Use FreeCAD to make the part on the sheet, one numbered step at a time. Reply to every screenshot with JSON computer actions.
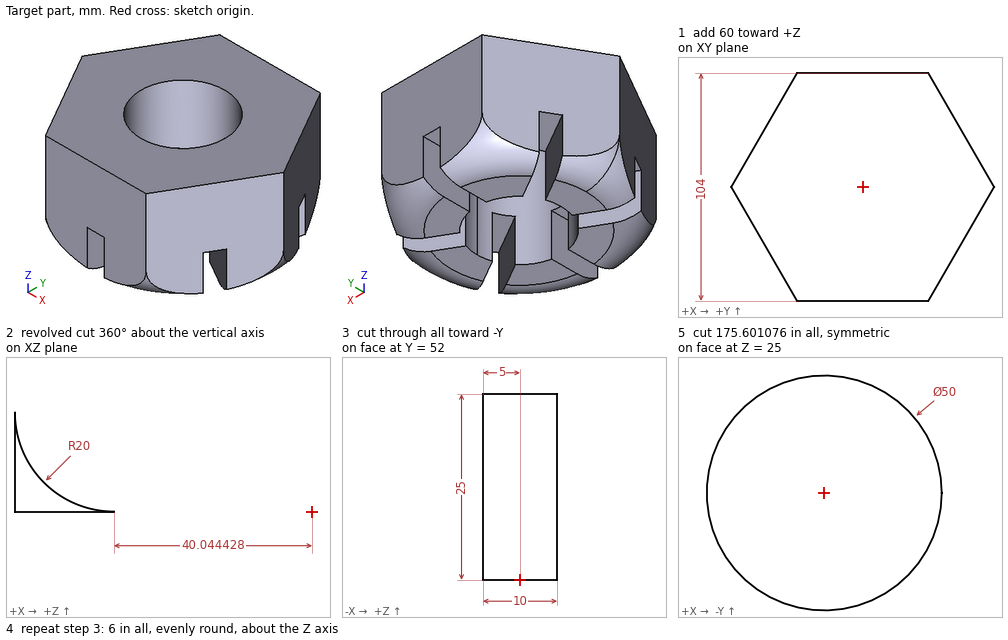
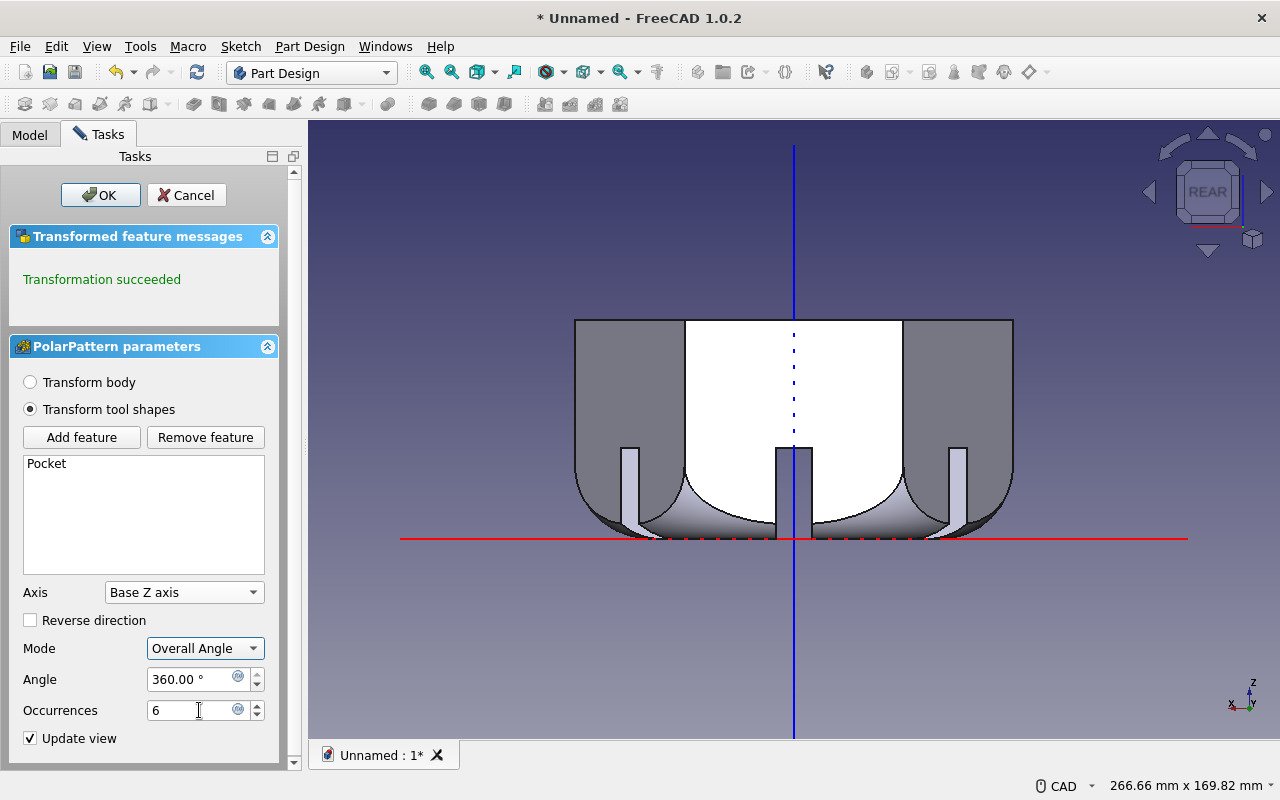
{"action": "left_click", "coordinate": [101, 195]}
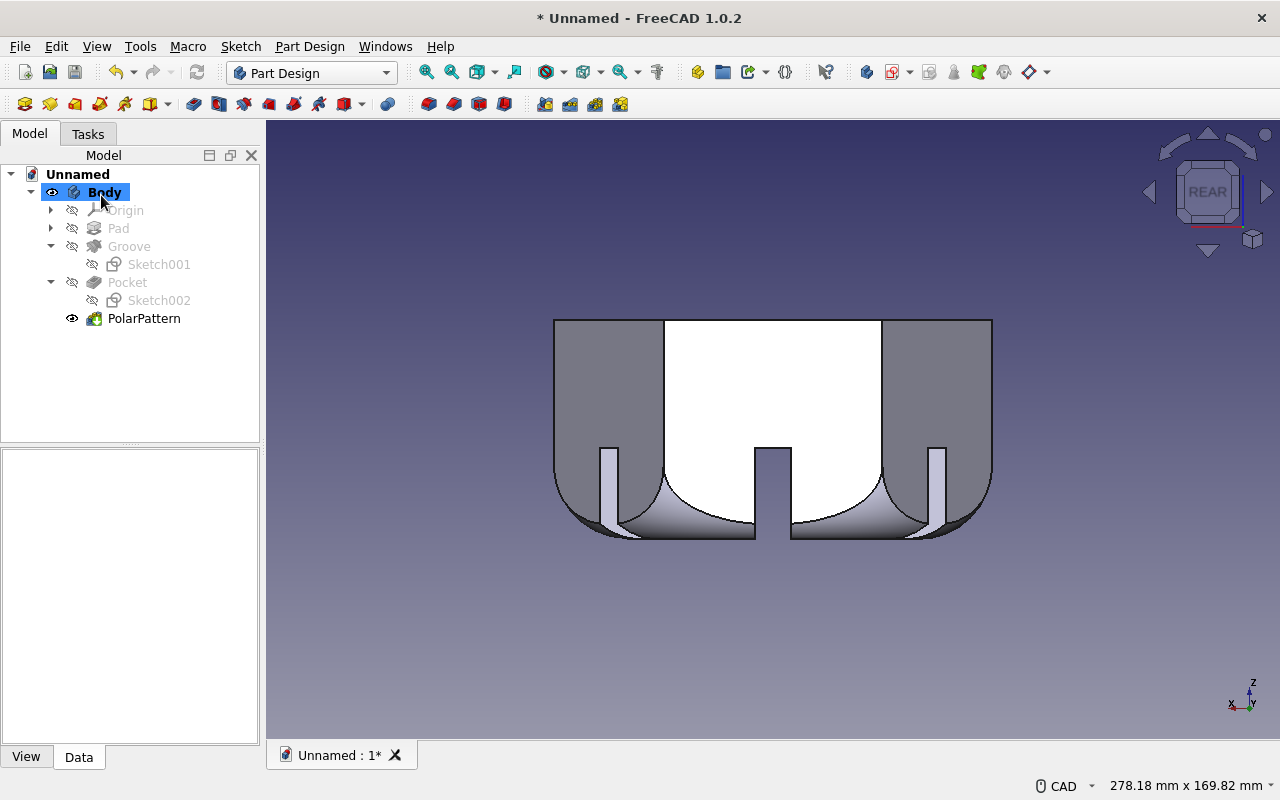
{"action": "left_click", "coordinate": [427, 72]}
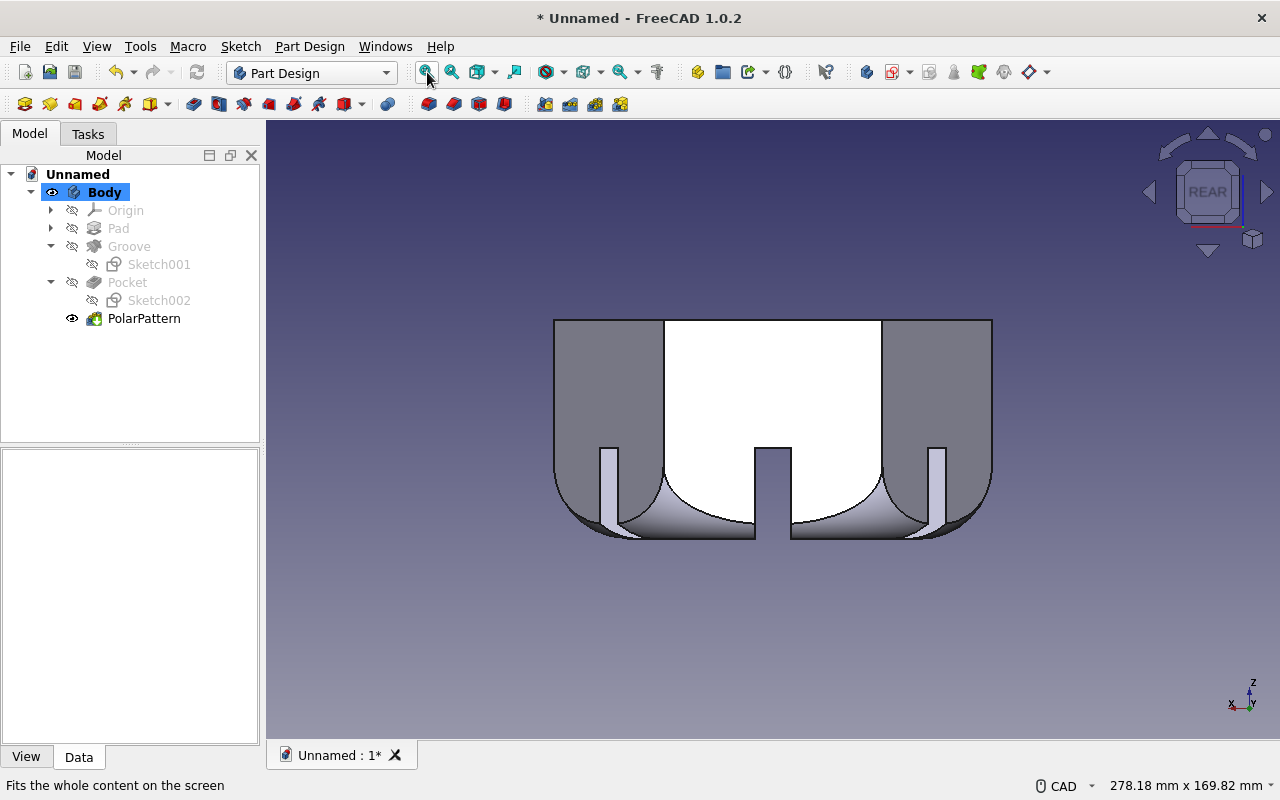
{"action": "key", "text": "5"}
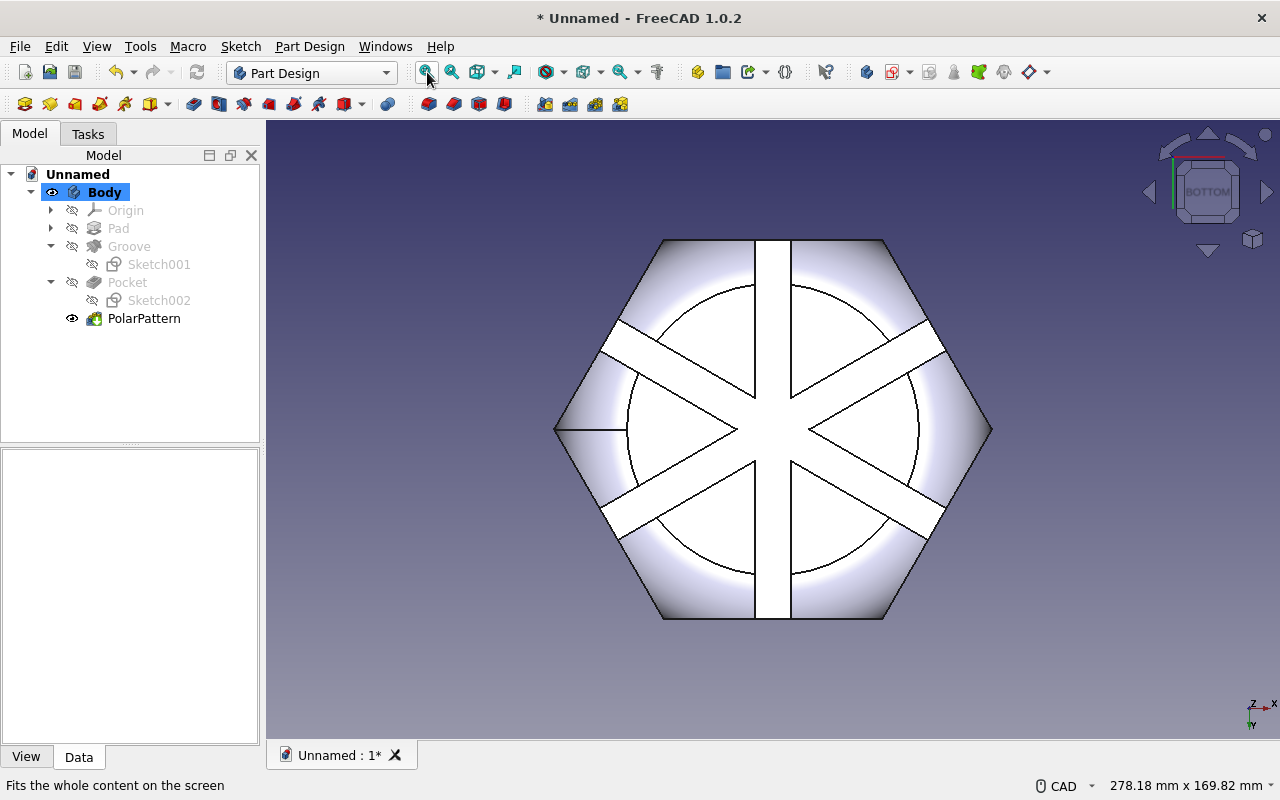
{"action": "left_click", "coordinate": [773, 428]}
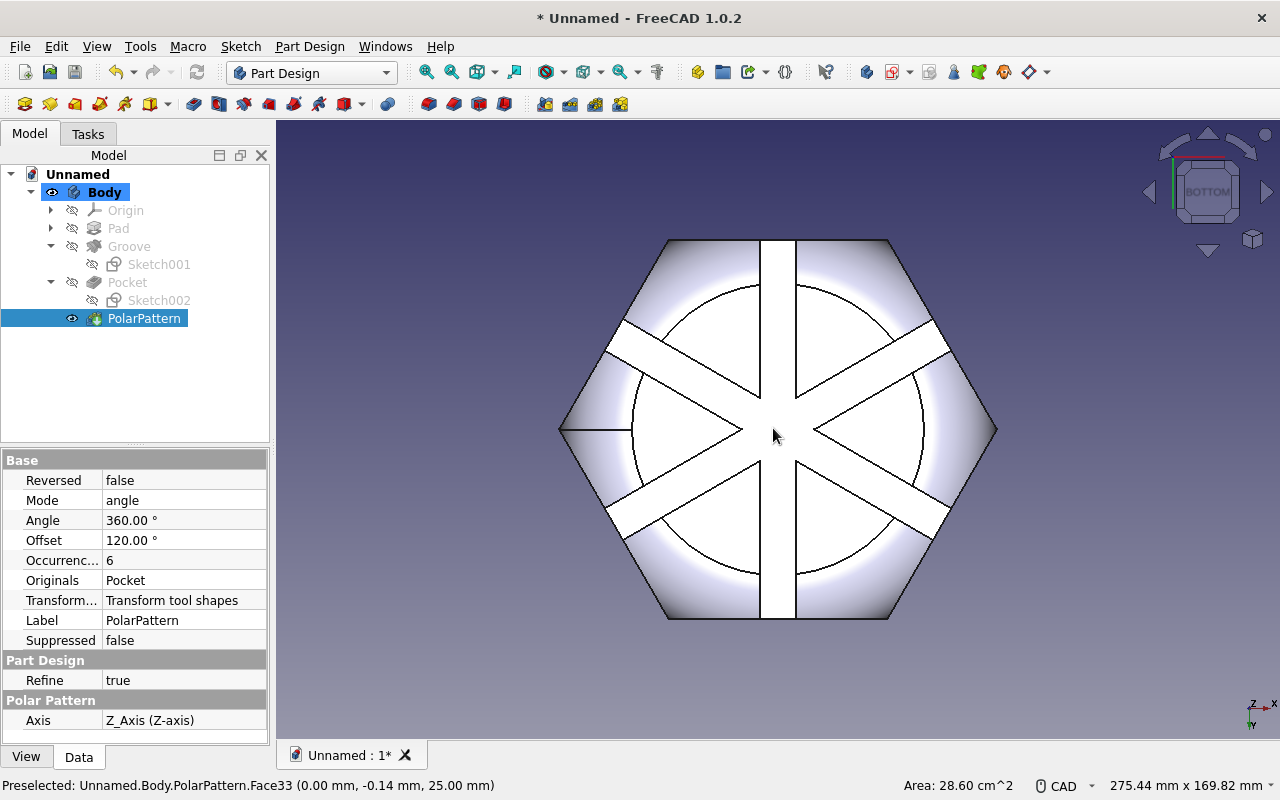
{"action": "left_click", "coordinate": [892, 72]}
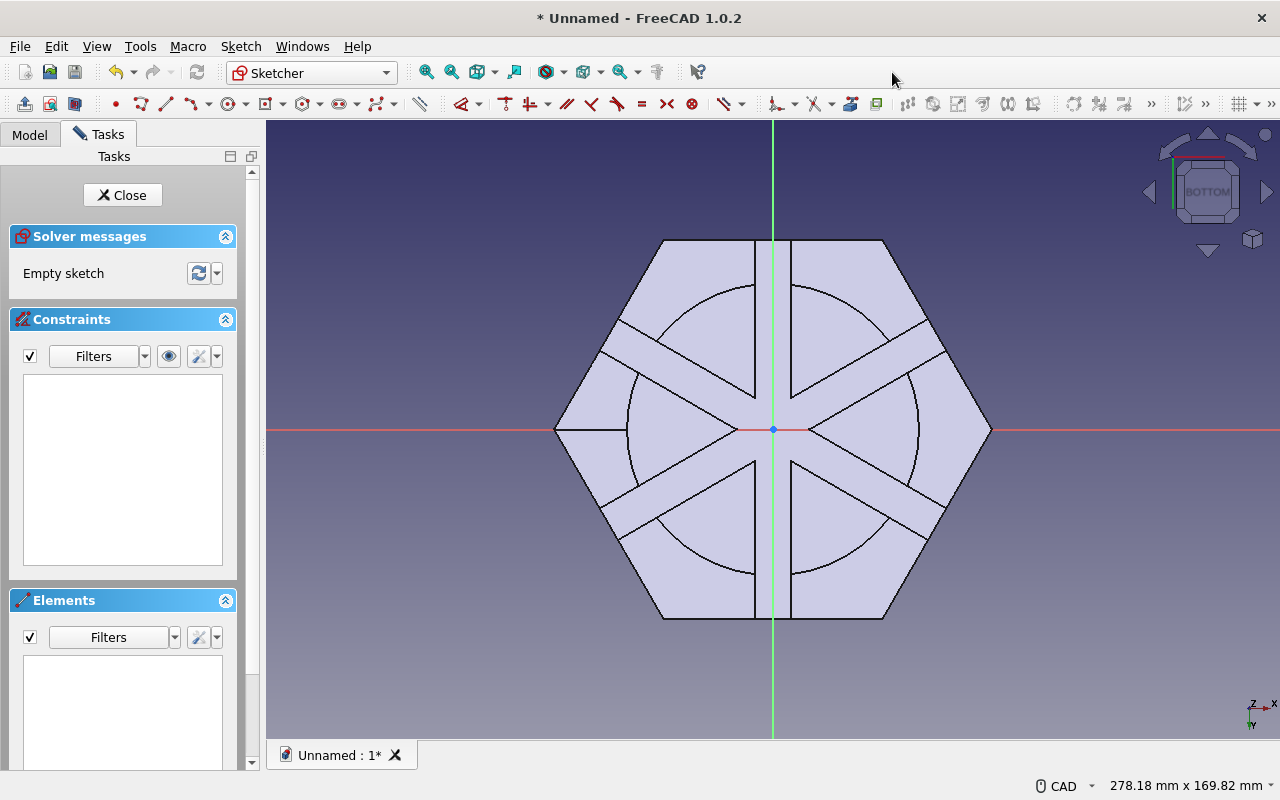
{"action": "key", "text": "q s"}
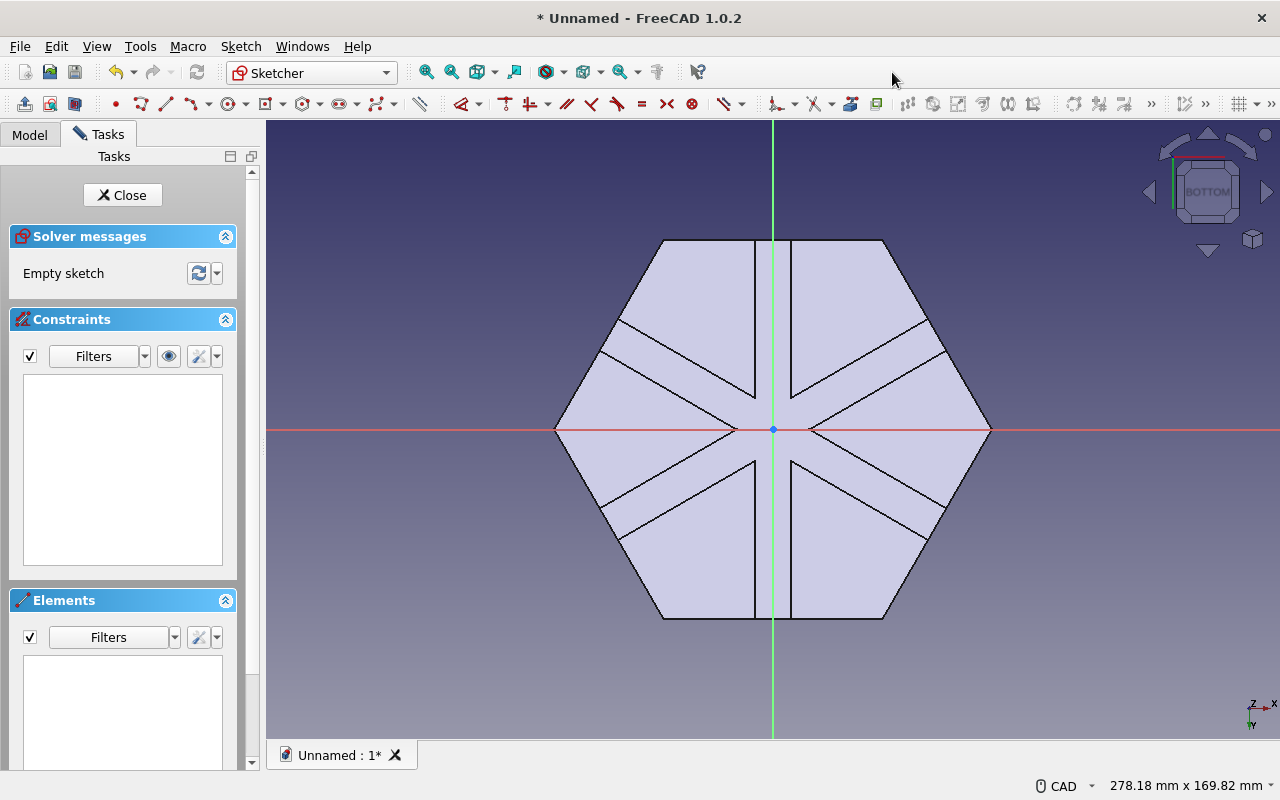
{"action": "scroll", "coordinate": [829, 430], "scroll_direction": "up", "scroll_amount": 4}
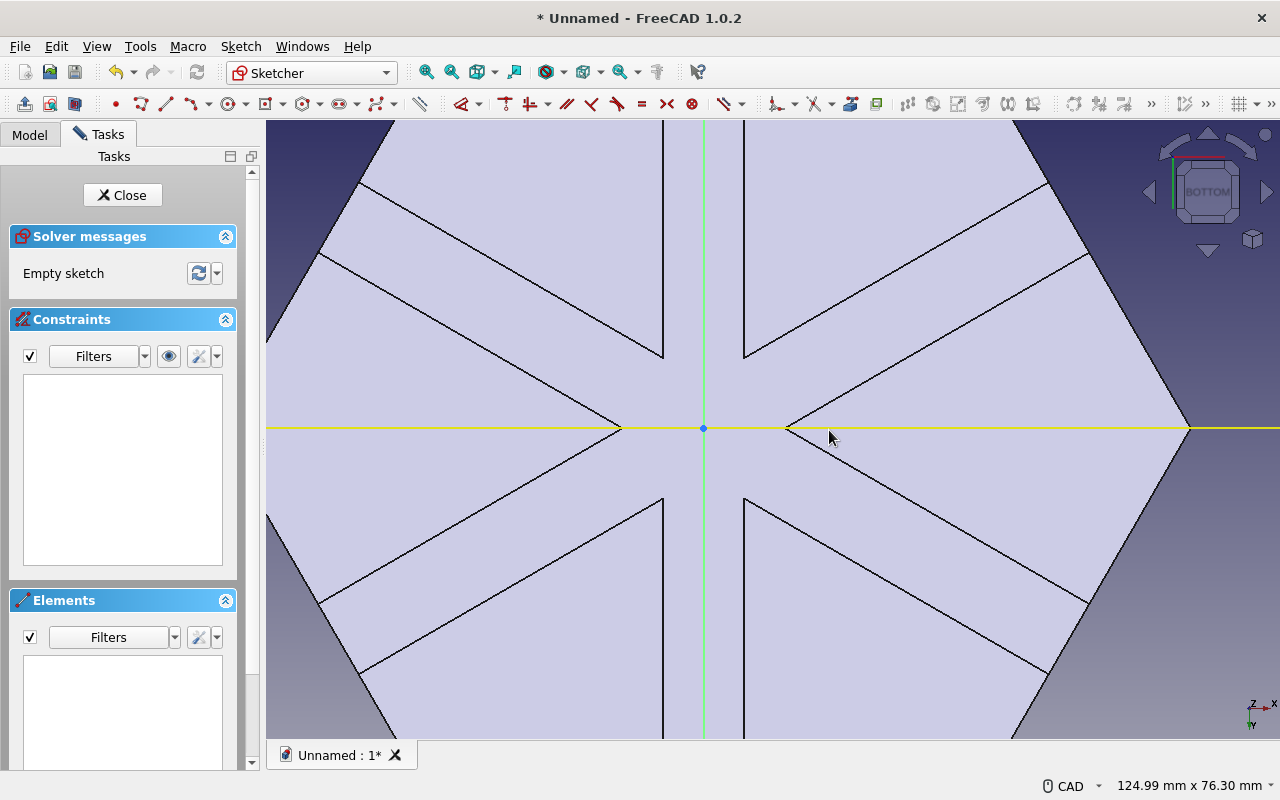
{"action": "left_click", "coordinate": [228, 104]}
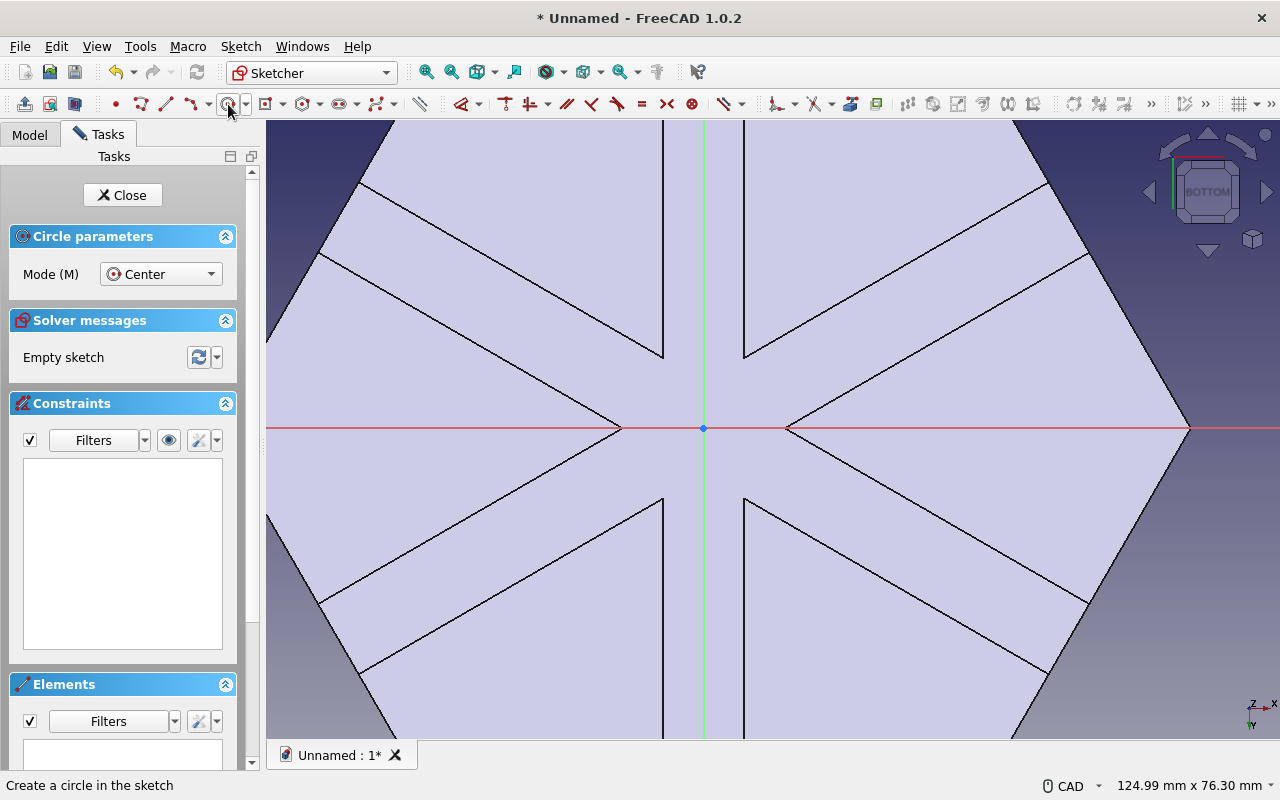
{"action": "left_click", "coordinate": [704, 428]}
{"action": "mouse_move", "coordinate": [847, 285]}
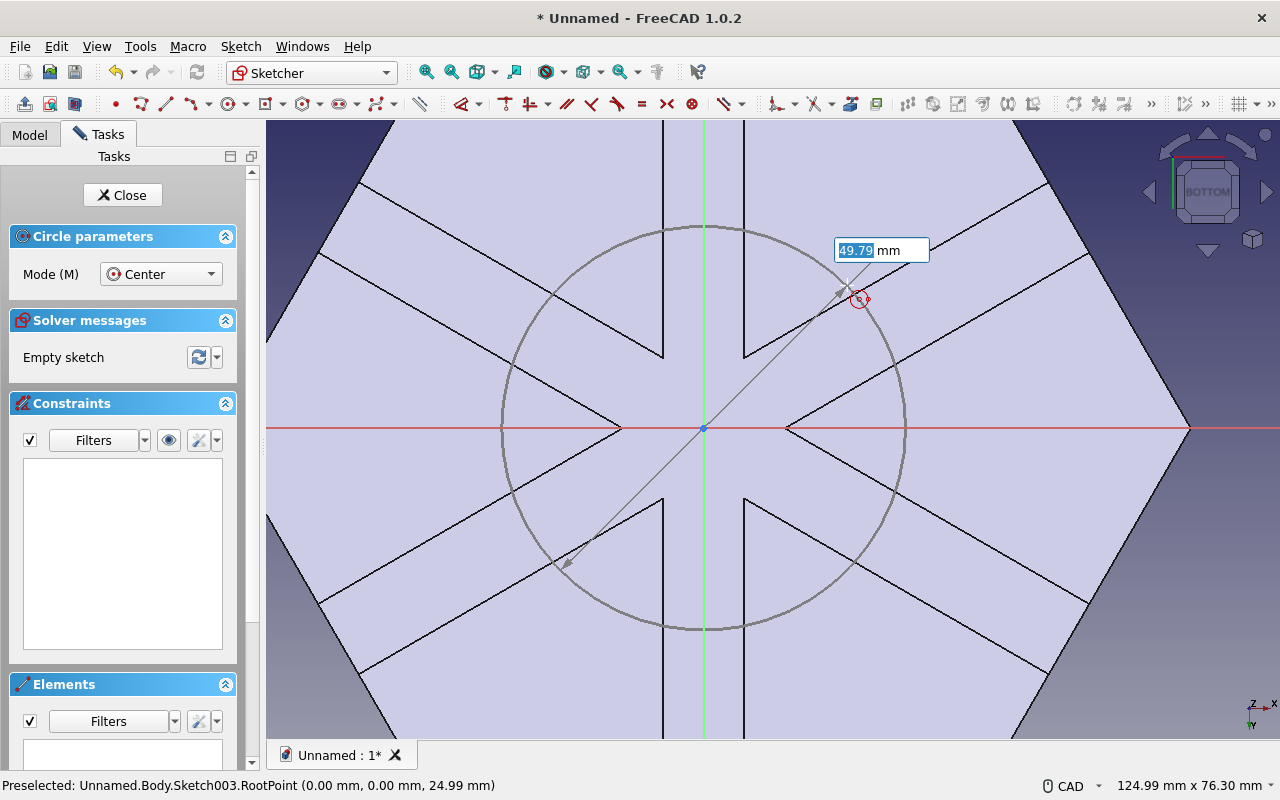
{"action": "type", "text": "50"}
{"action": "key", "text": "Return"}
{"action": "key", "text": "Escape"}